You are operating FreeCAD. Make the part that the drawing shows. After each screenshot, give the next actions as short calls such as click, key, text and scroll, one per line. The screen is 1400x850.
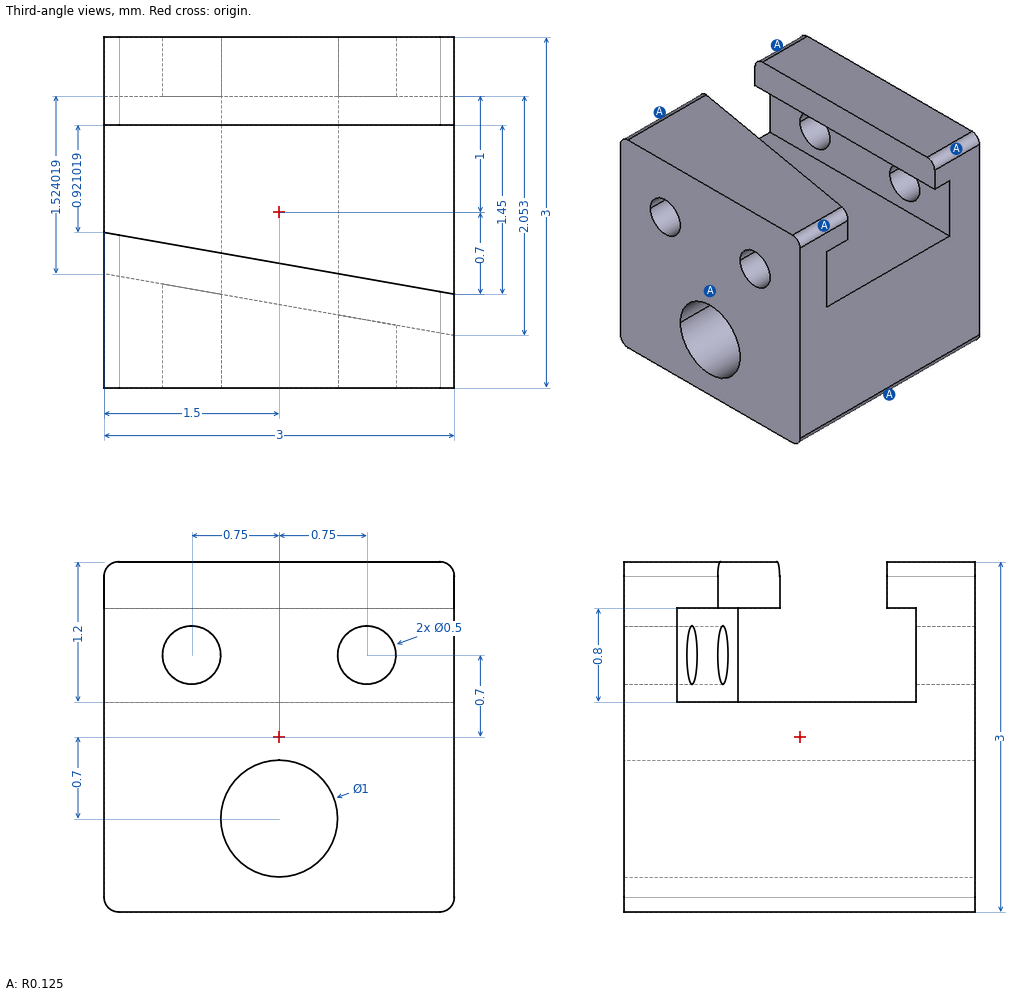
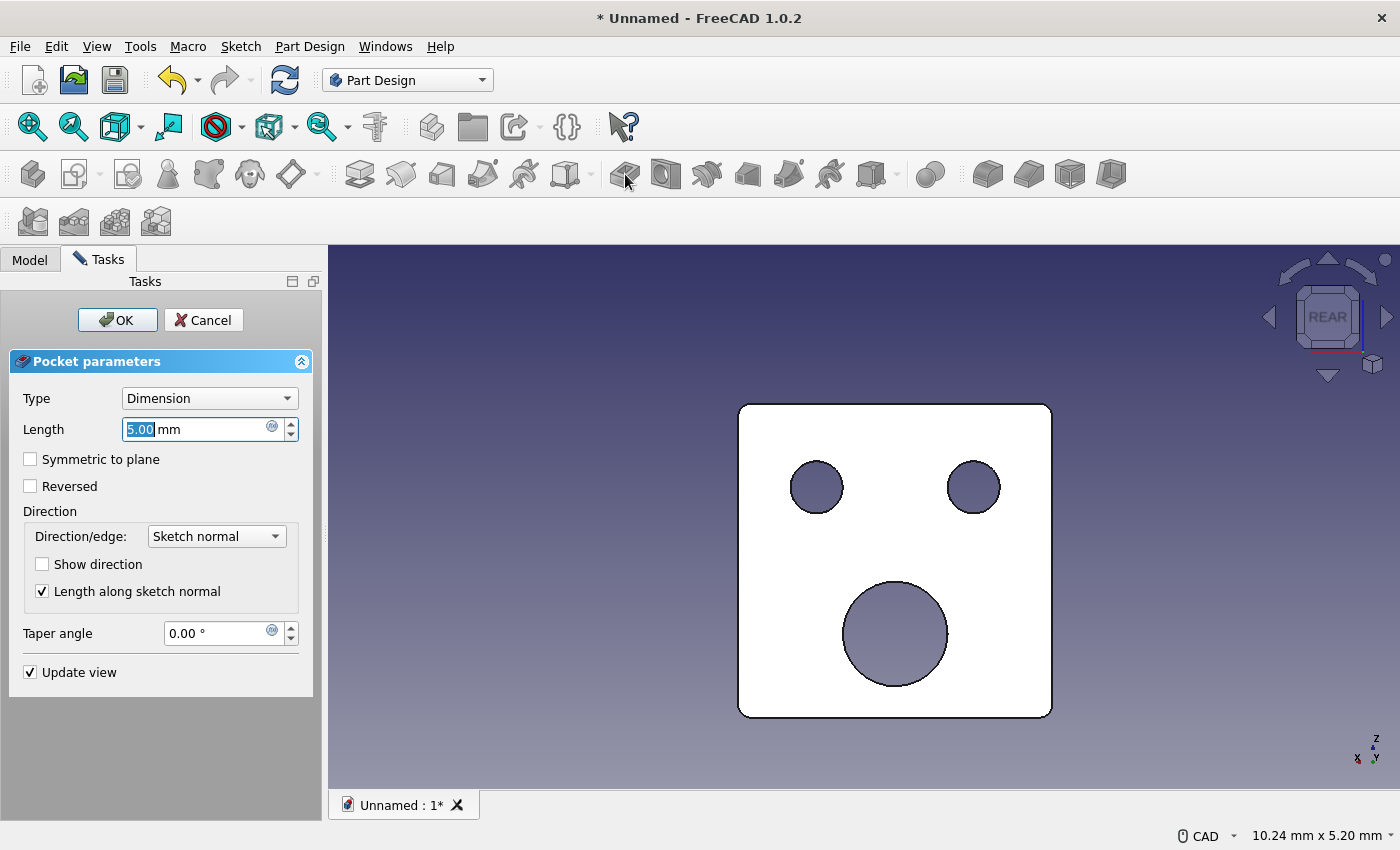
click(210, 398)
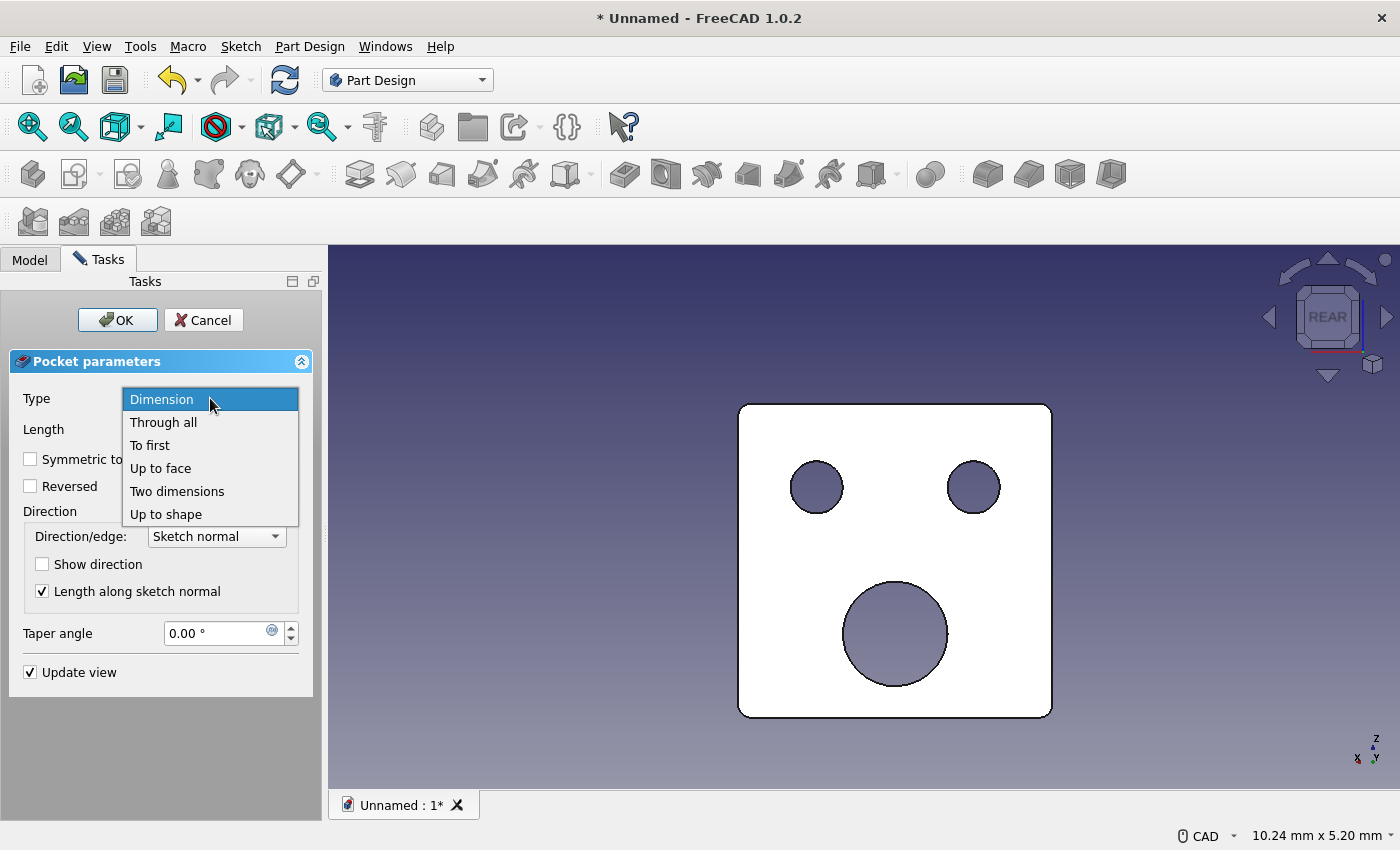
click(208, 422)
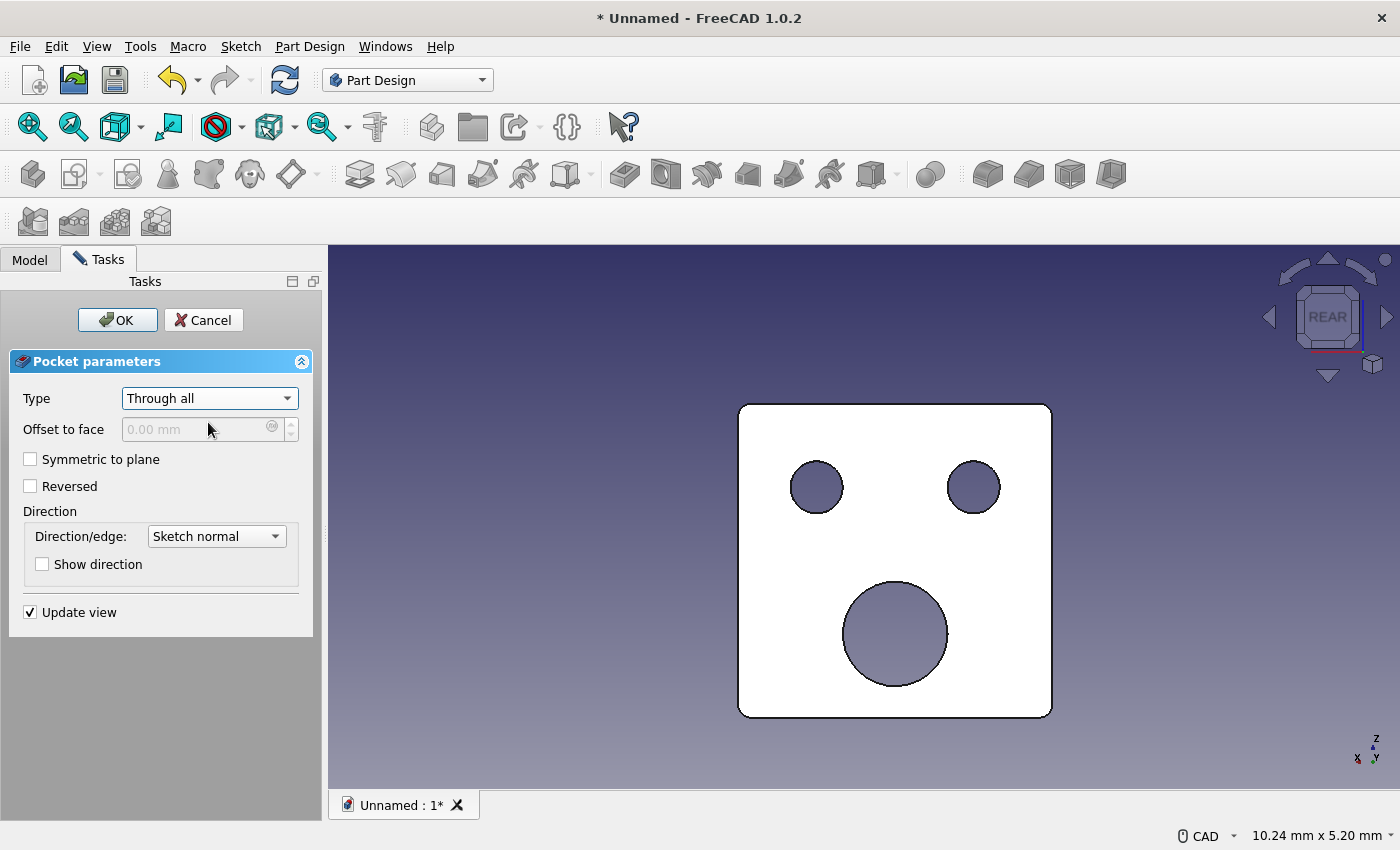
click(118, 320)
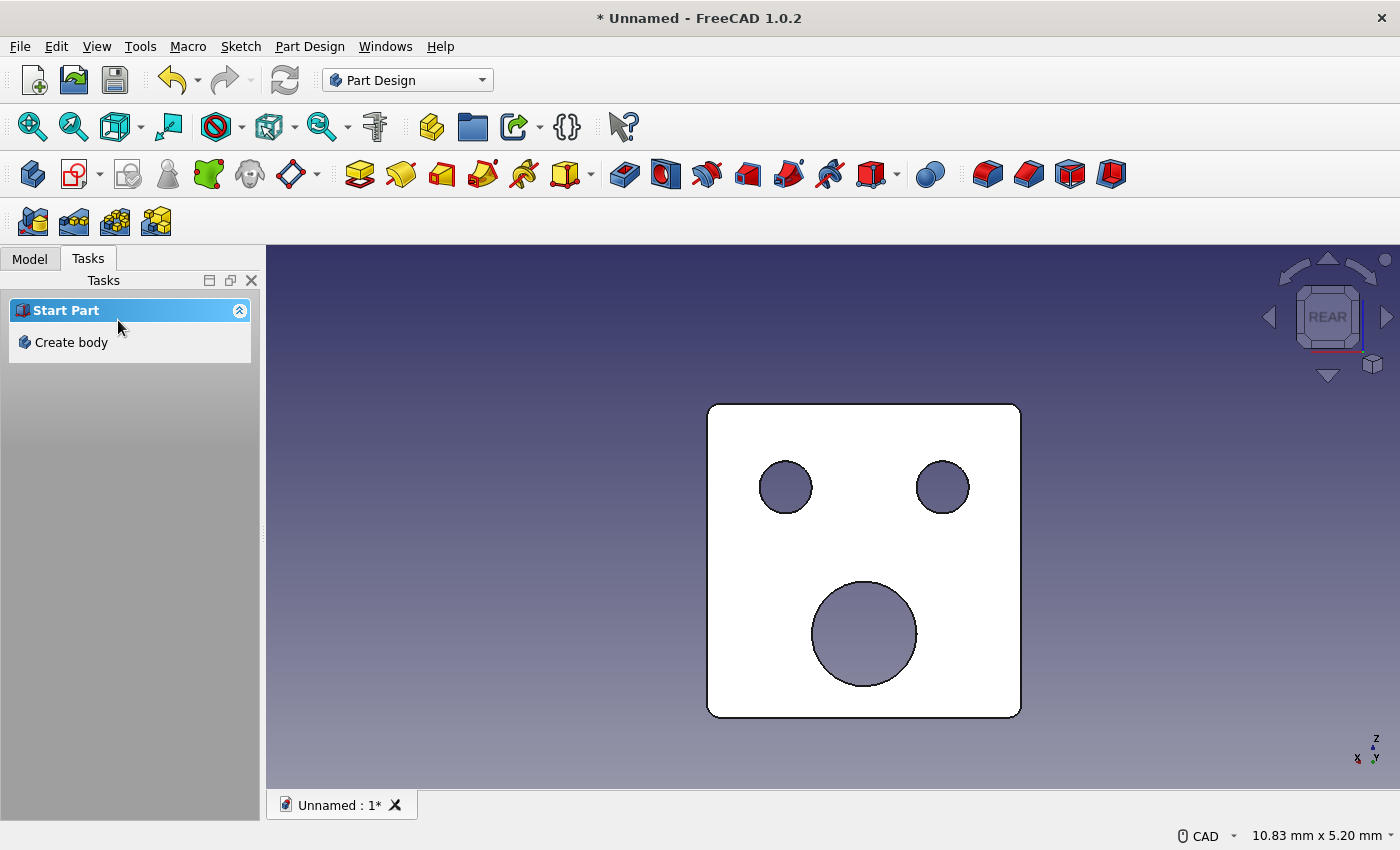
key(0)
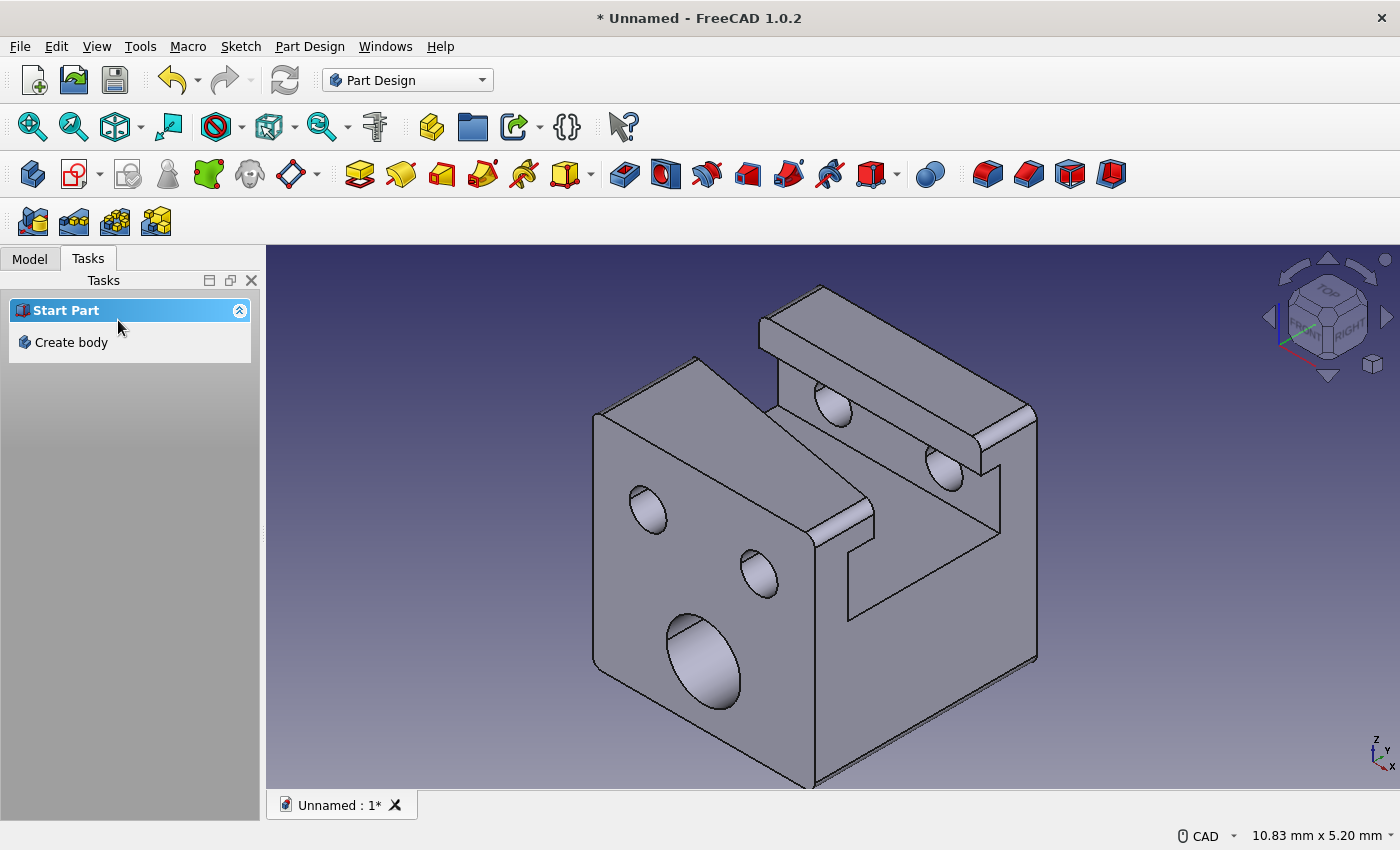
click(33, 128)